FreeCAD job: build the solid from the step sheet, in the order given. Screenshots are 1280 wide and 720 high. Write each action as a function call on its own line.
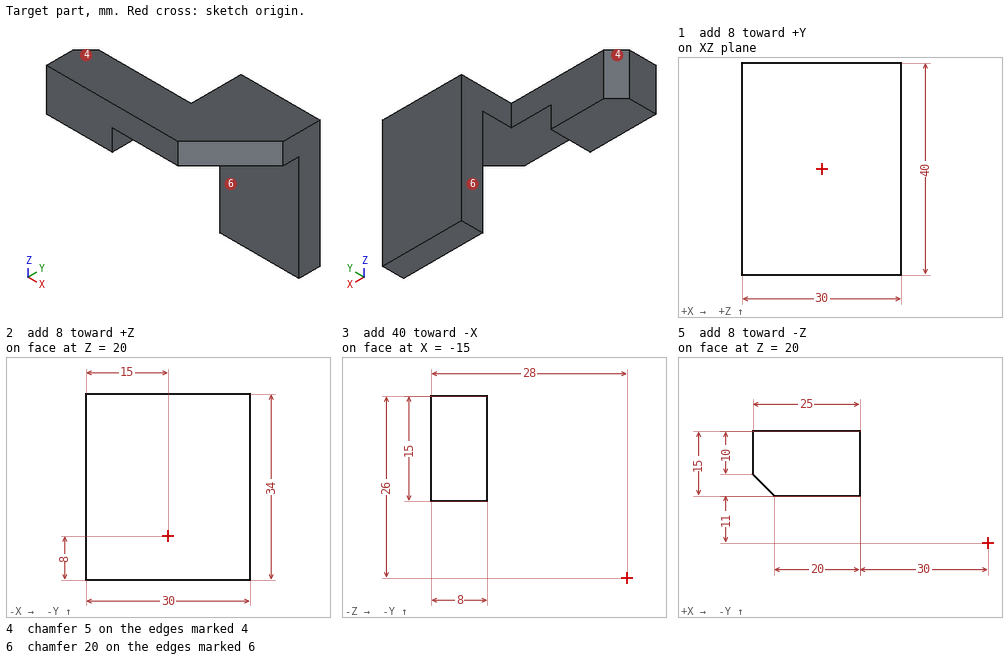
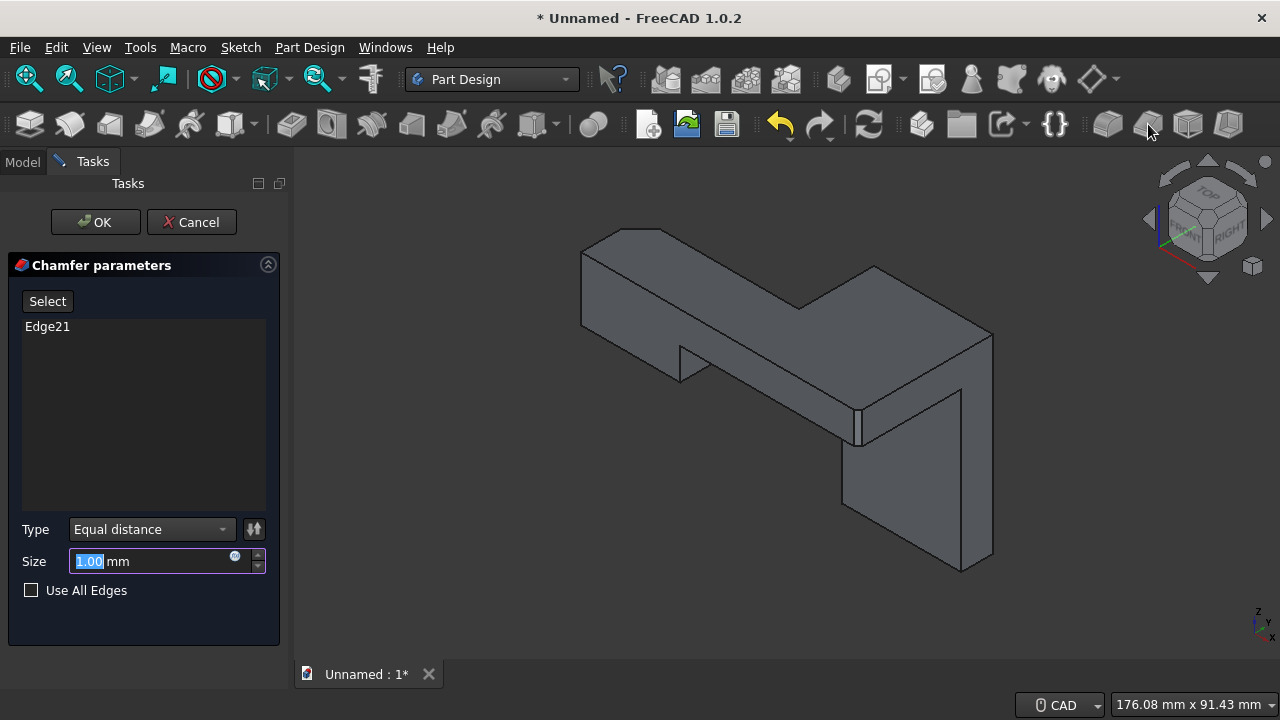
text(20)
key(Tab)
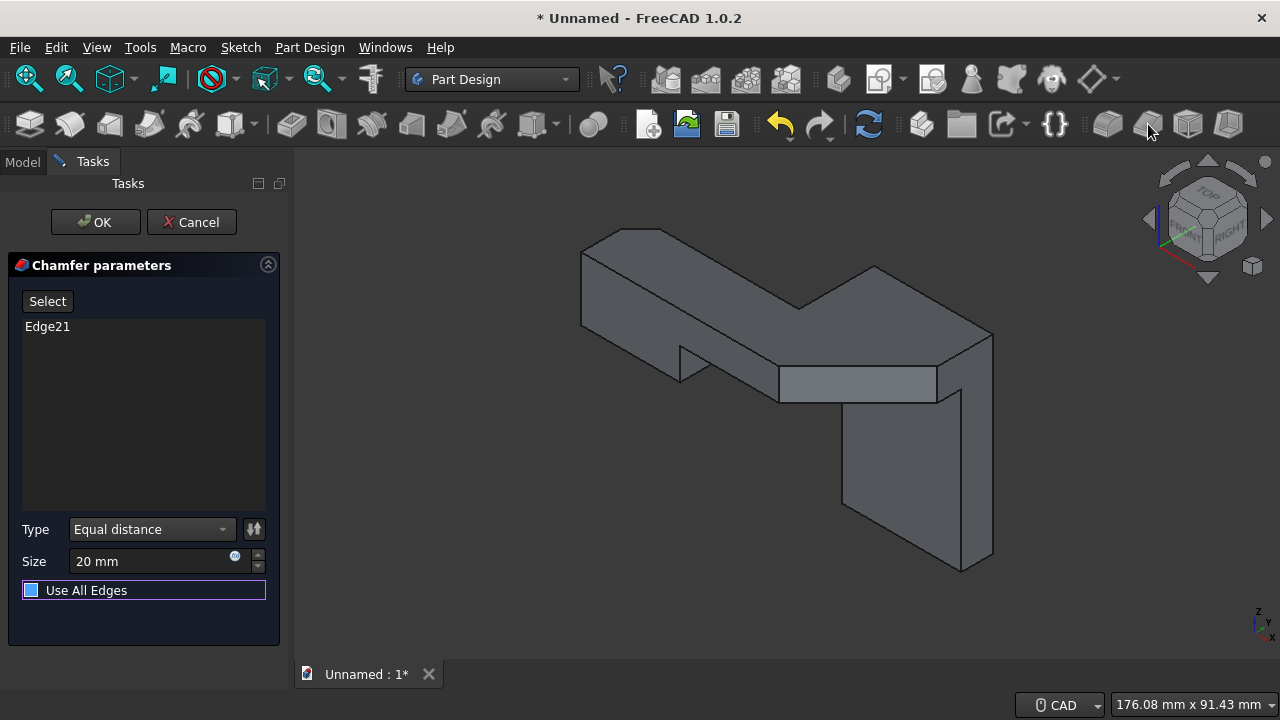
click(96, 222)